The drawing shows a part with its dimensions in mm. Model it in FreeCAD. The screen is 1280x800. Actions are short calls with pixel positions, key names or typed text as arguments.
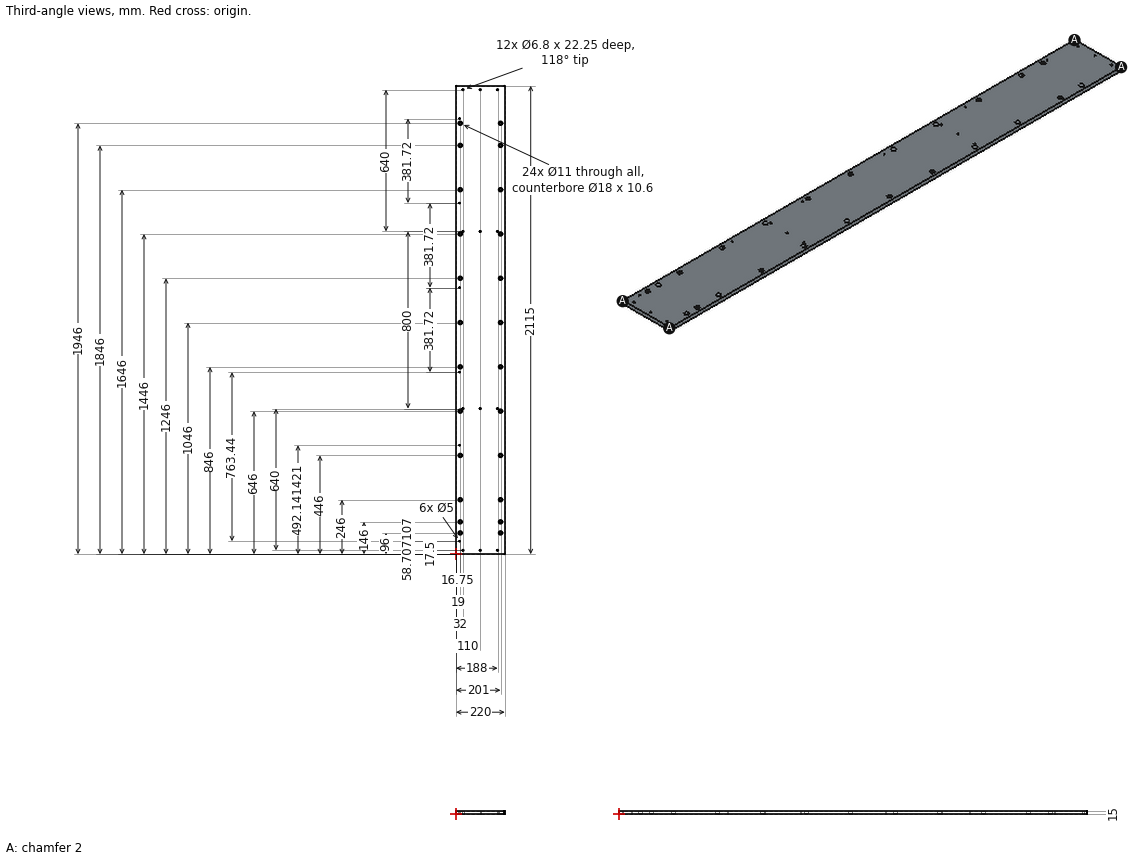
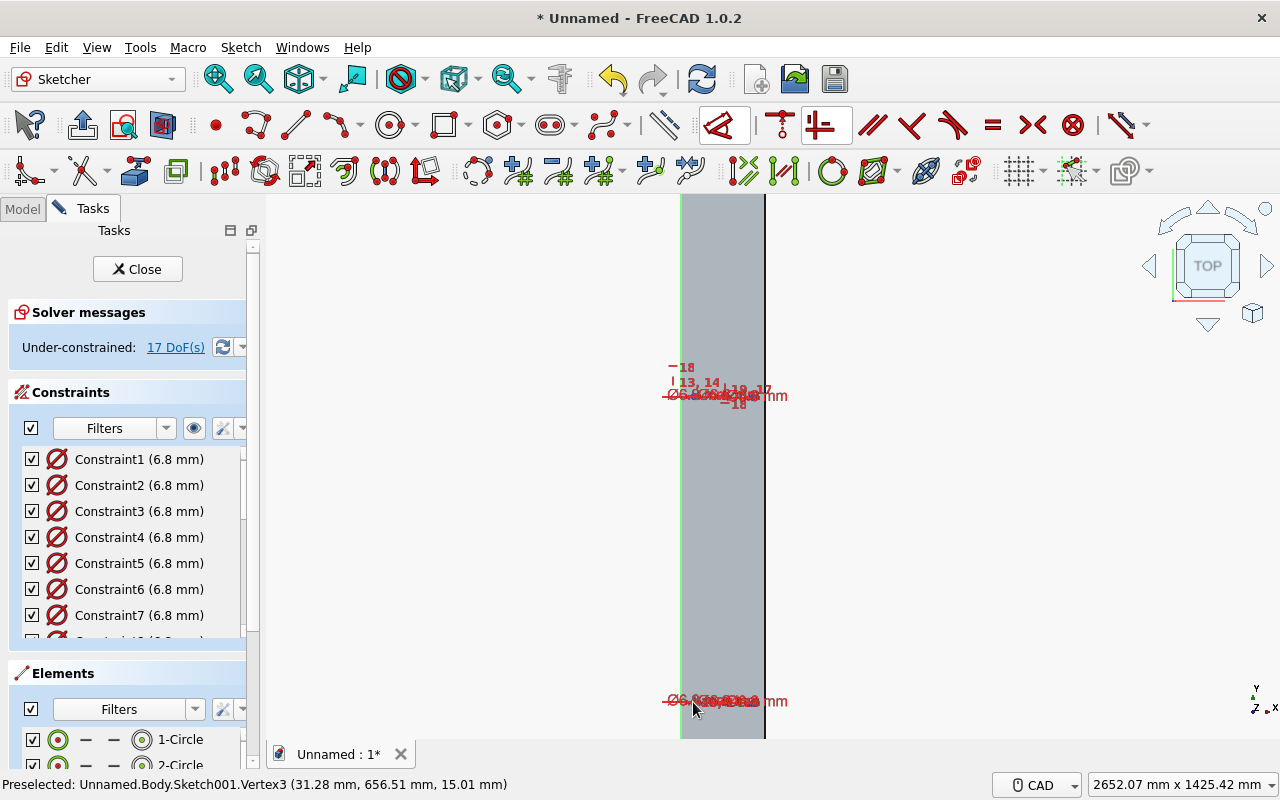
click(724, 703)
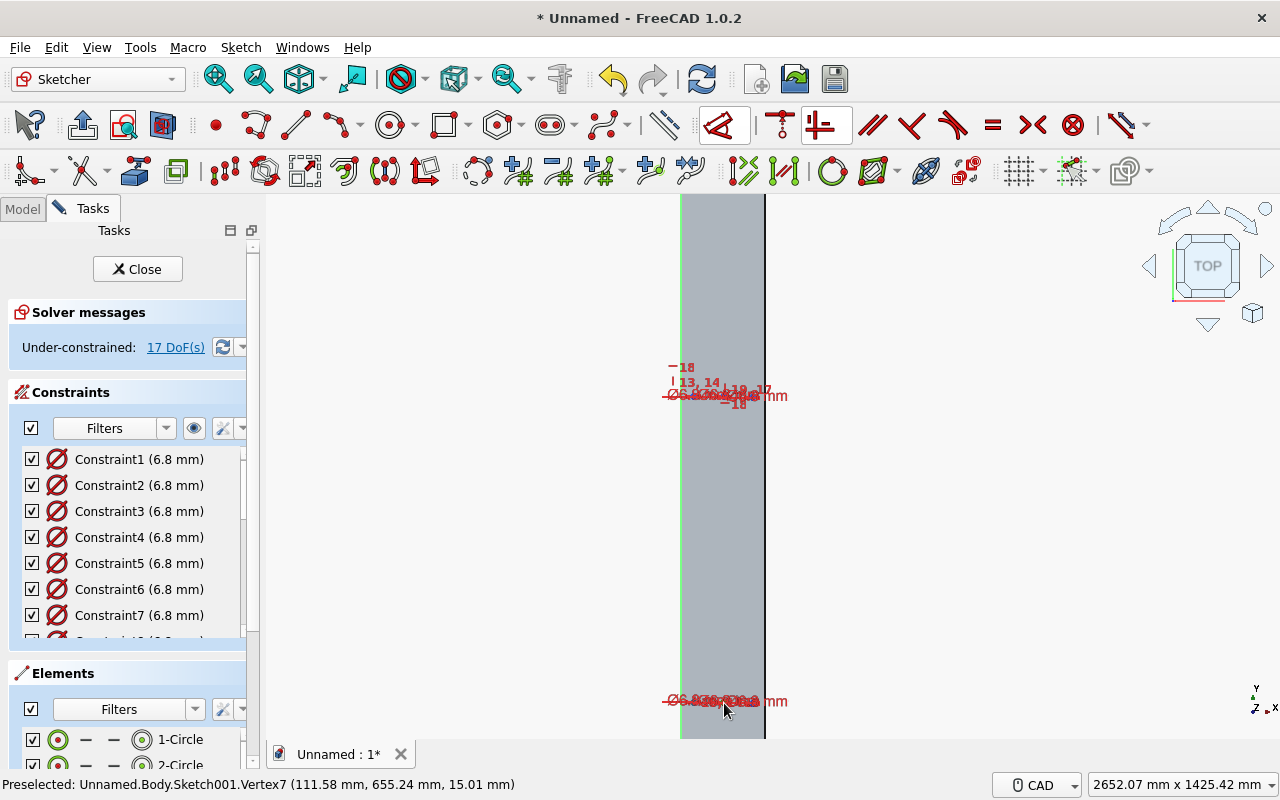
click(846, 126)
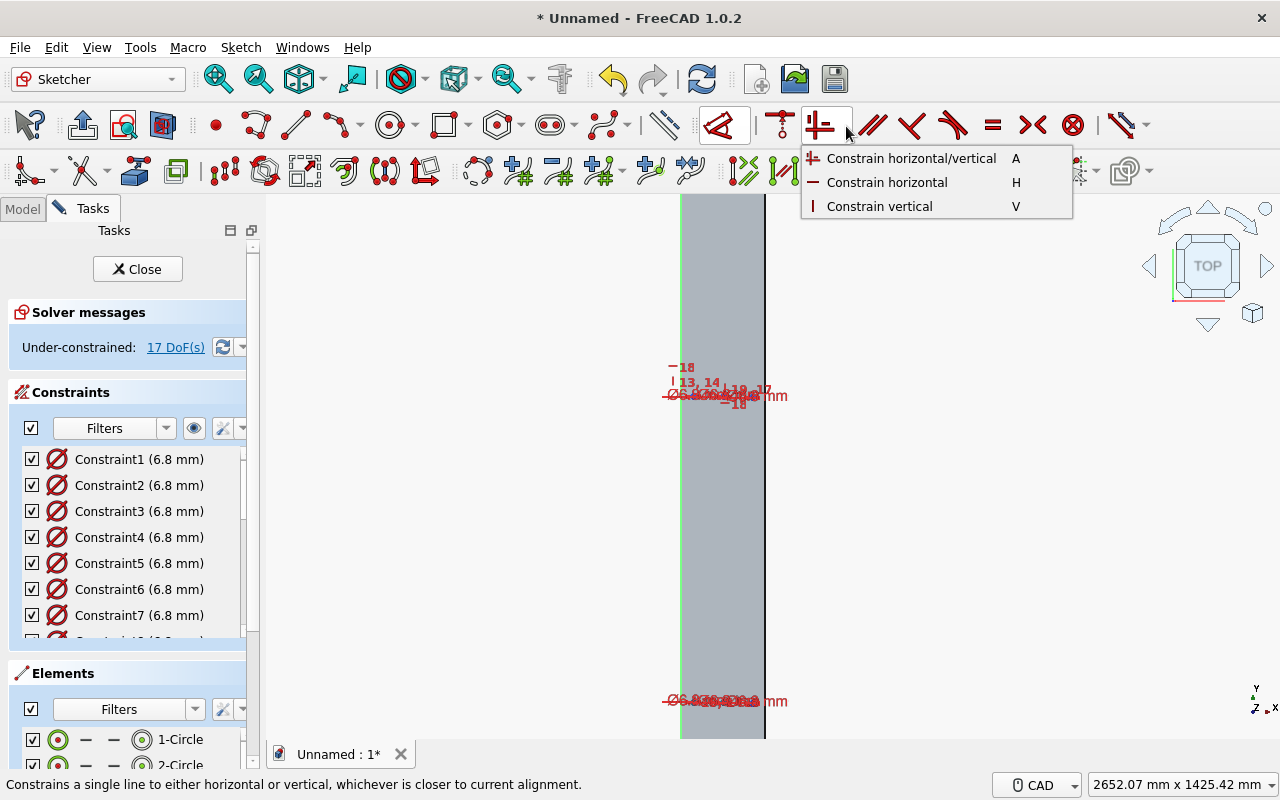
click(937, 182)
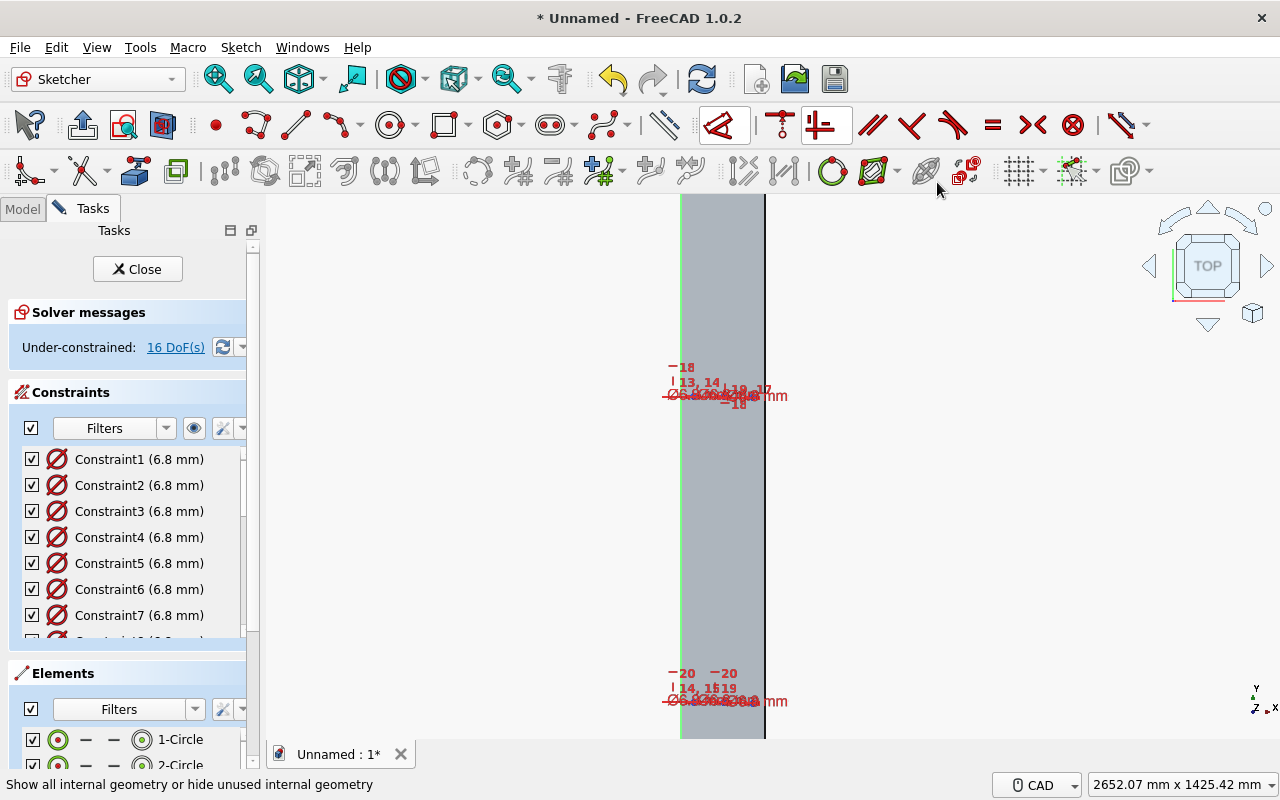
click(724, 702)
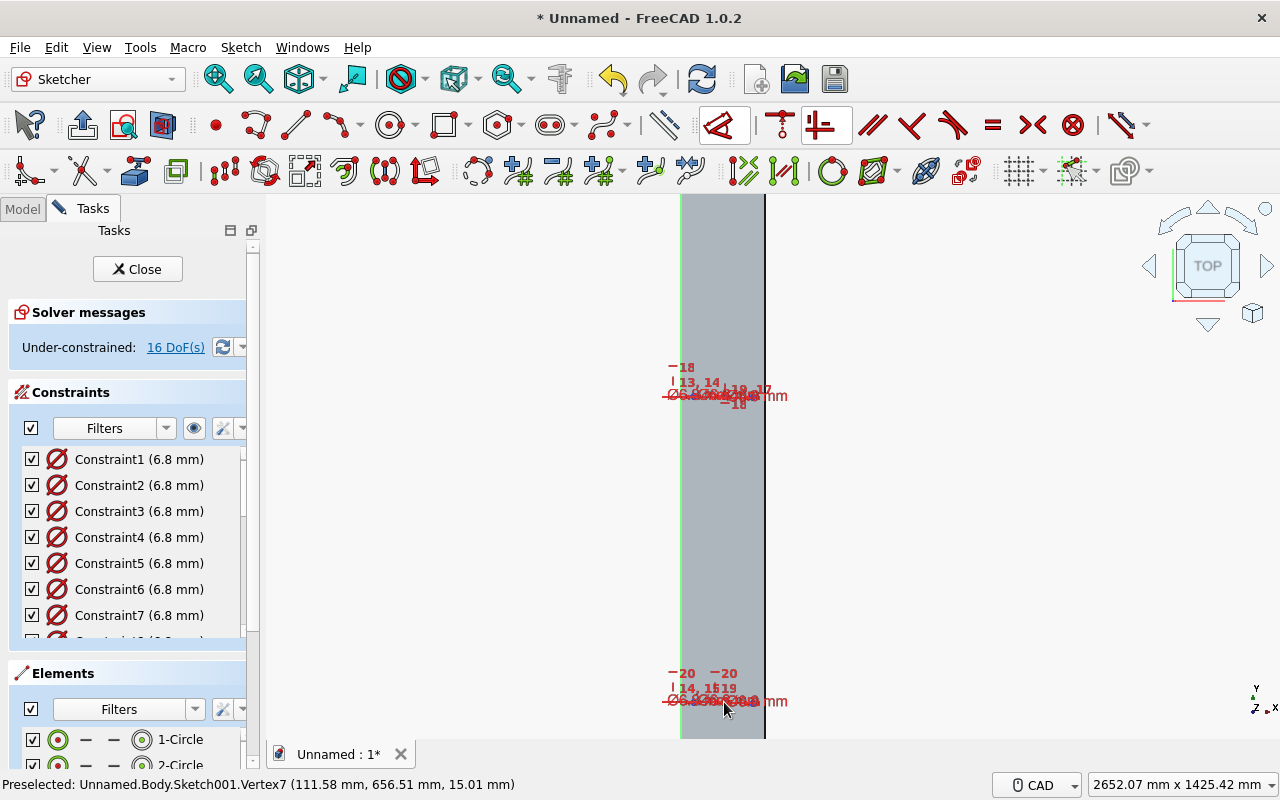
scroll(694, 397, down, 4)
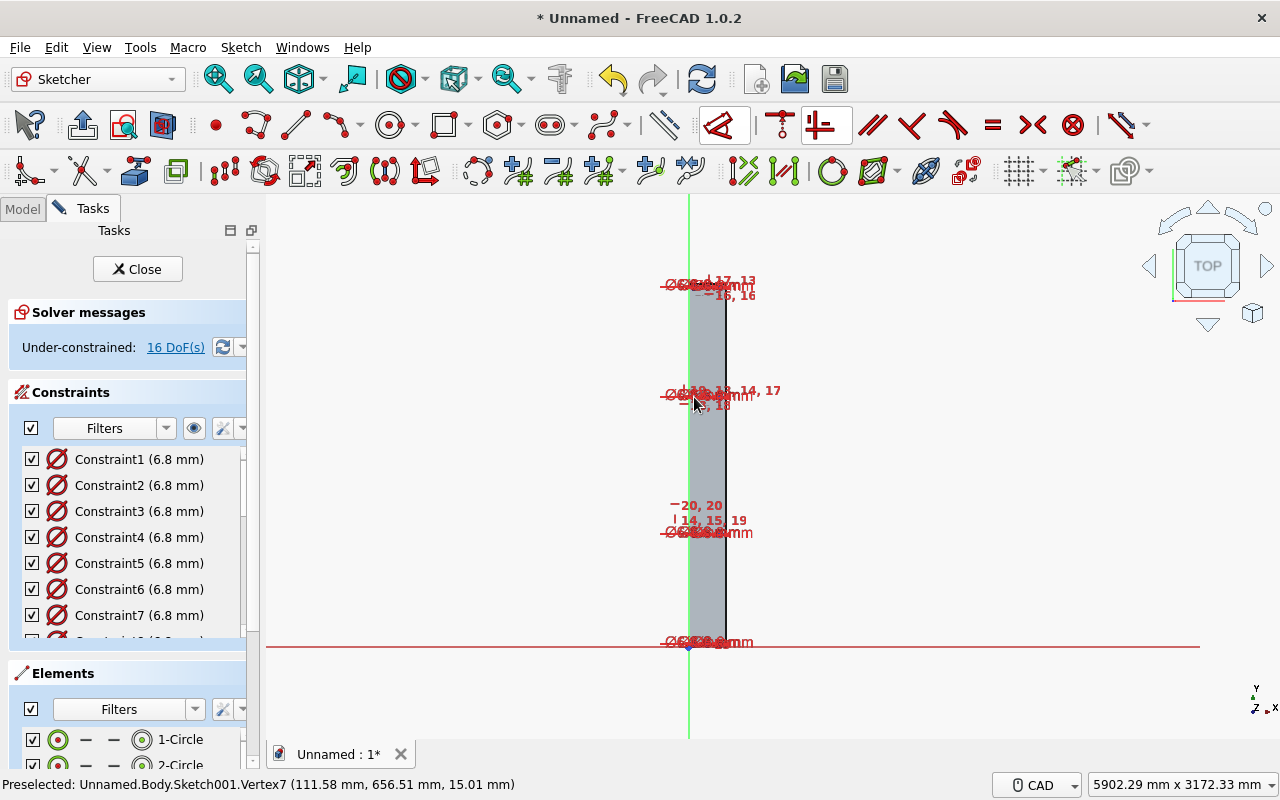
scroll(707, 644, up, 4)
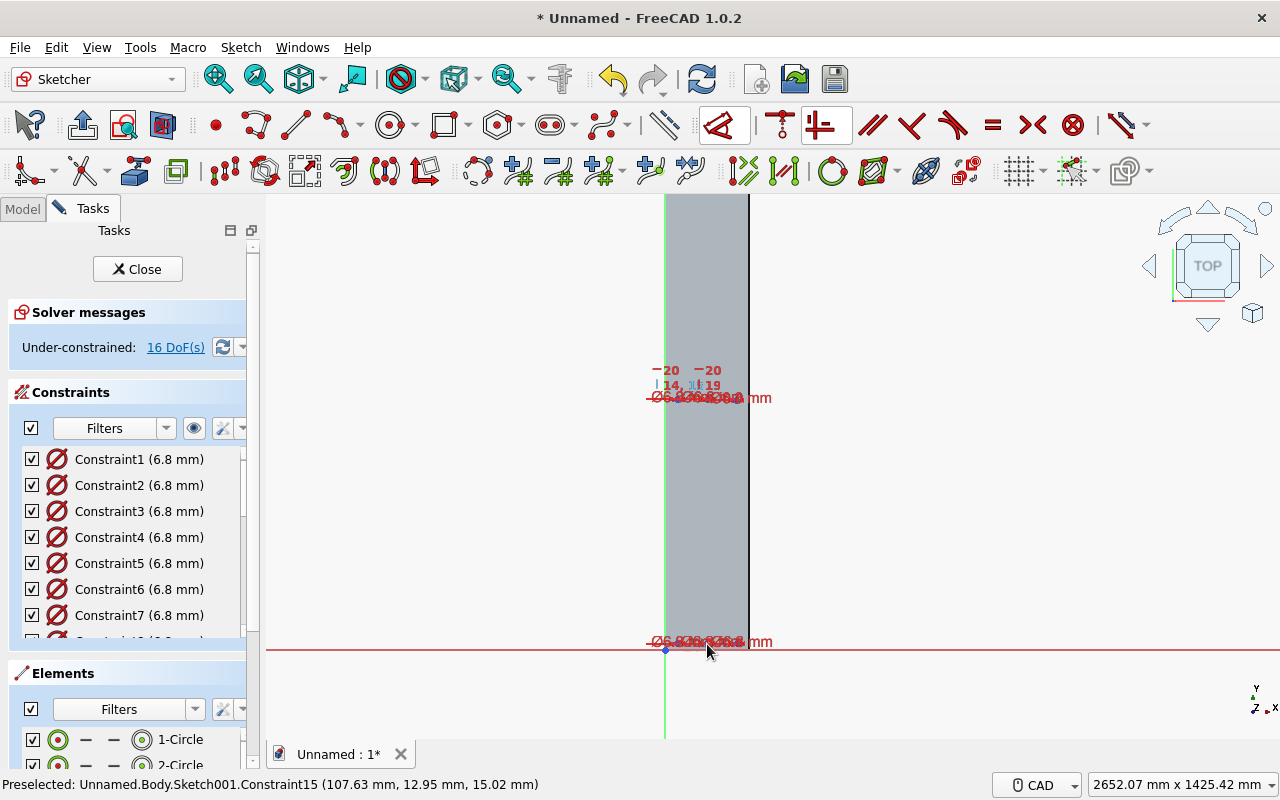
scroll(707, 644, up, 4)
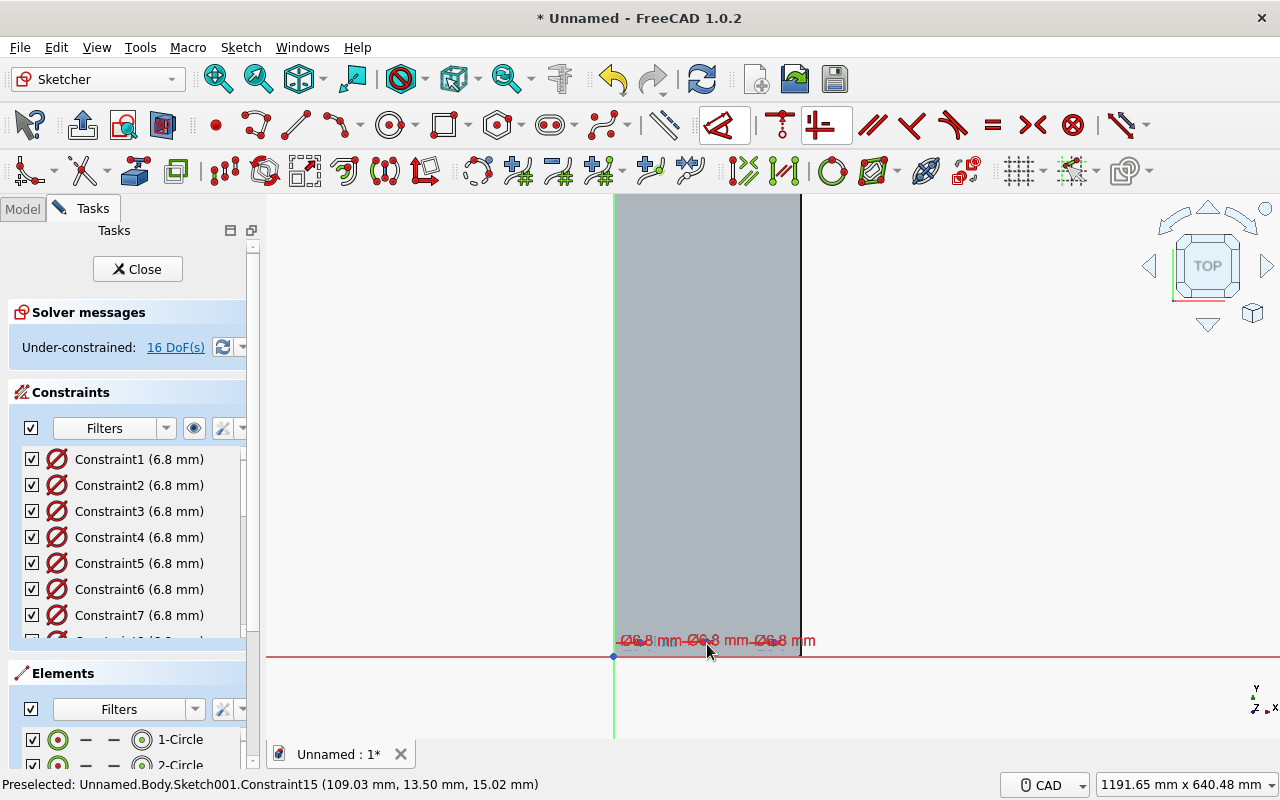
click(707, 642)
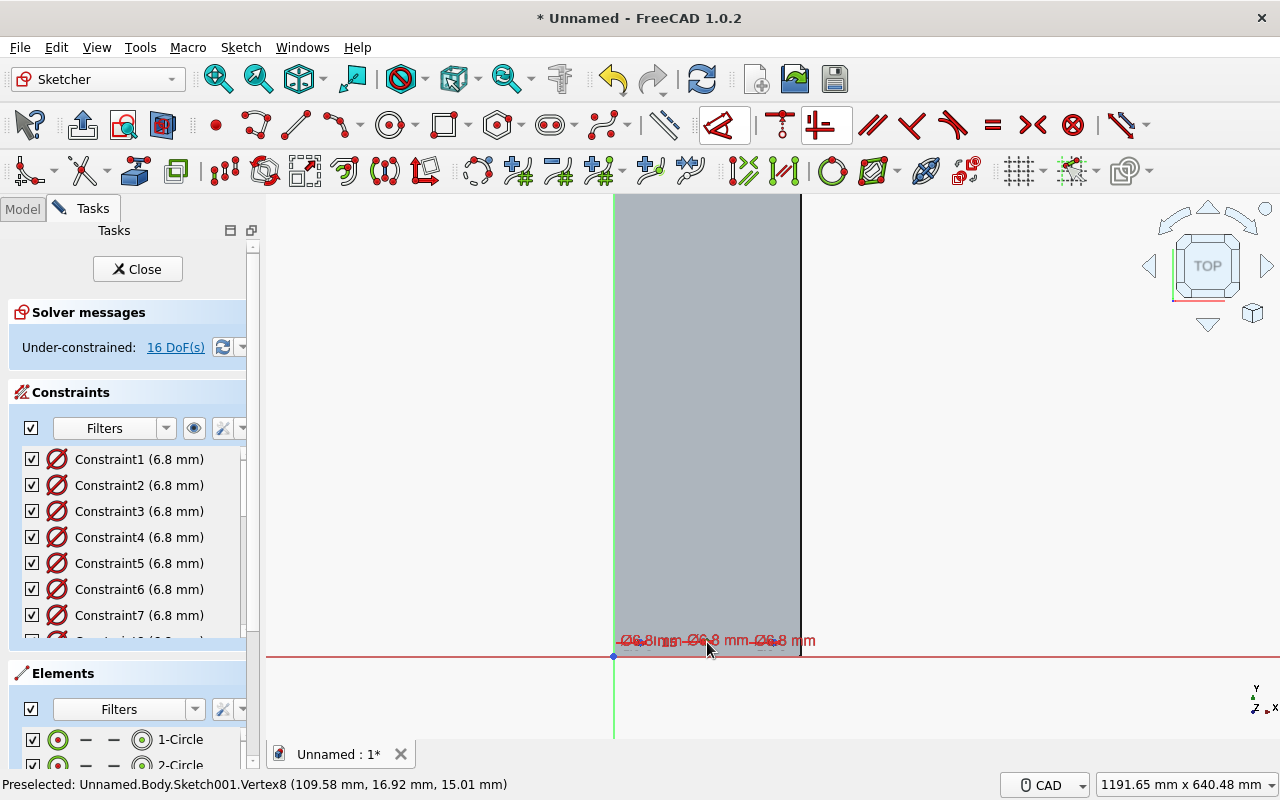
key(v)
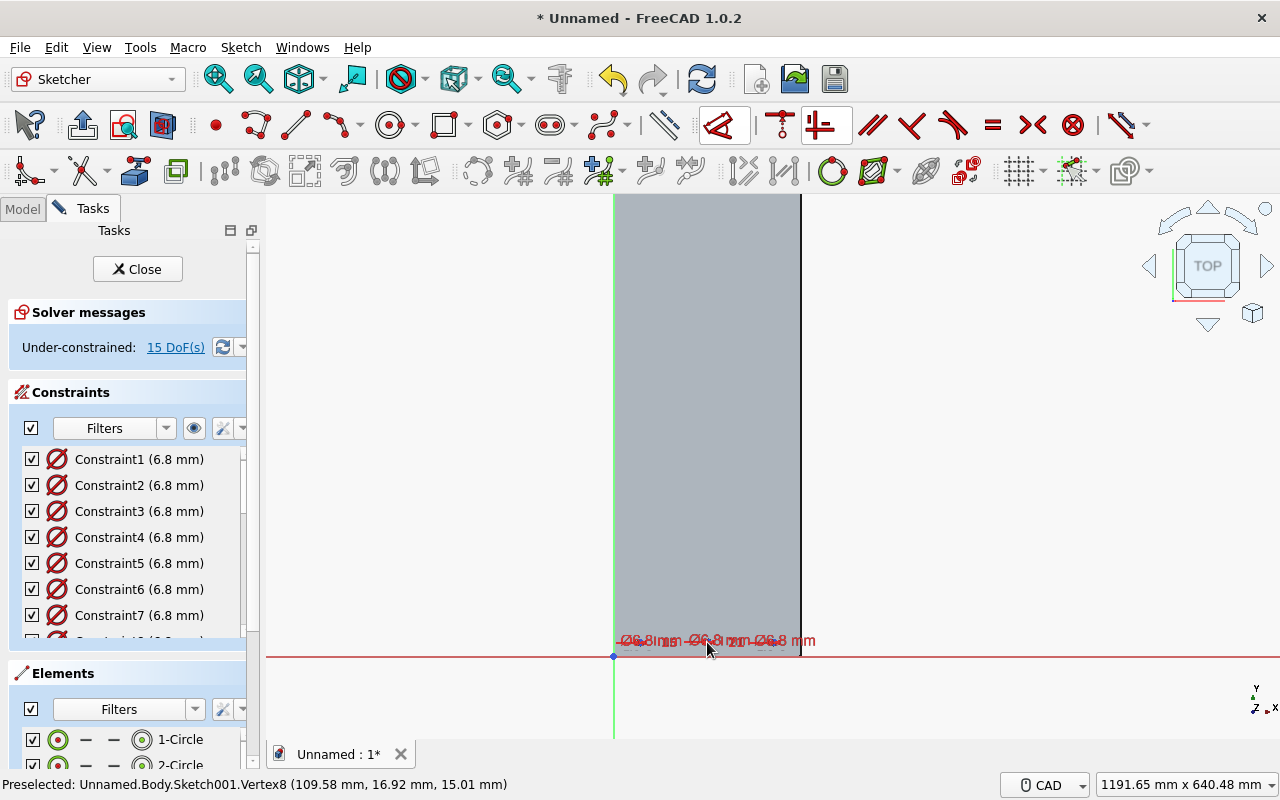
click(640, 643)